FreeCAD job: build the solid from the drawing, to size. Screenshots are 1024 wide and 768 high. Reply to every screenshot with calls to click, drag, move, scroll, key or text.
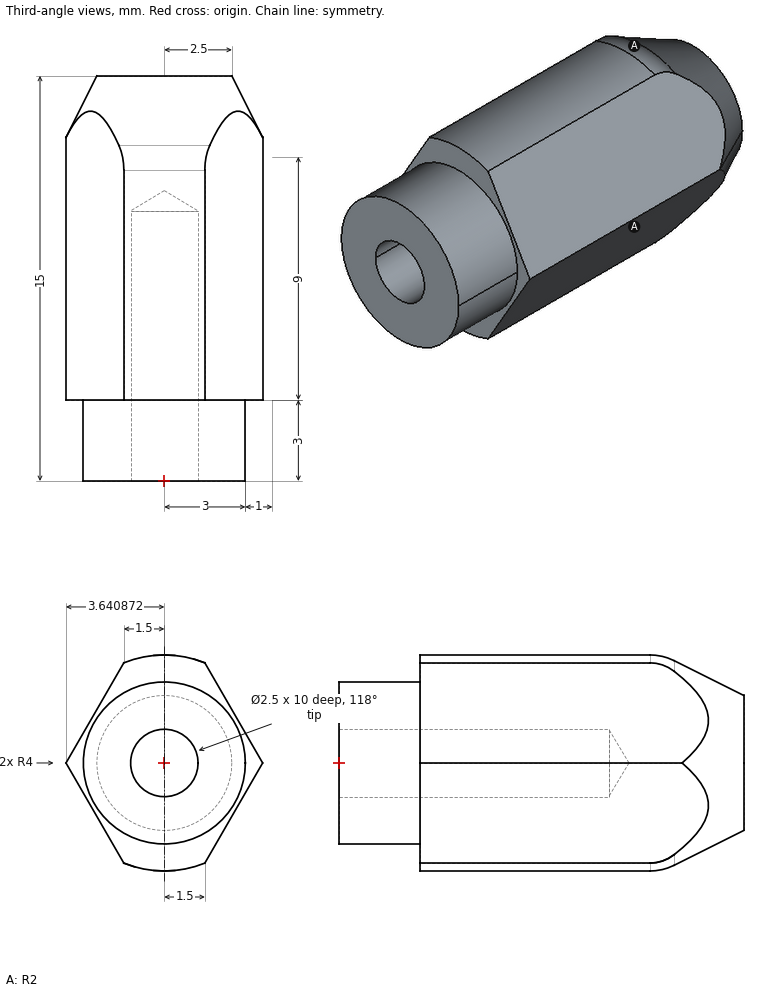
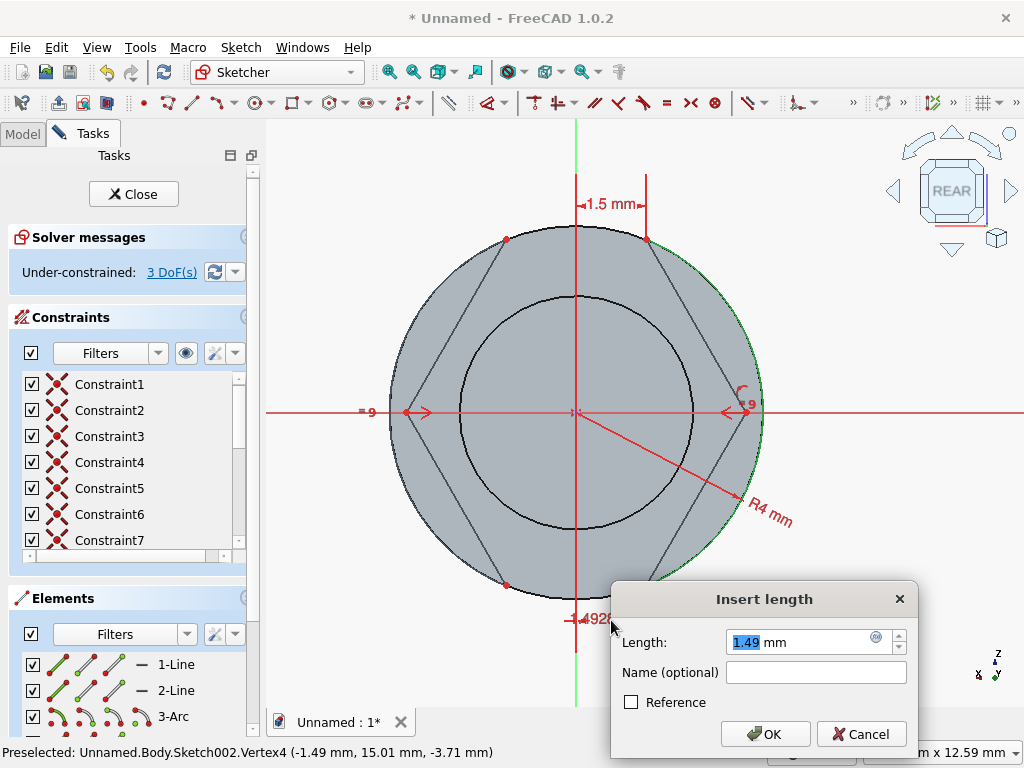
text(1.5)
key(Return)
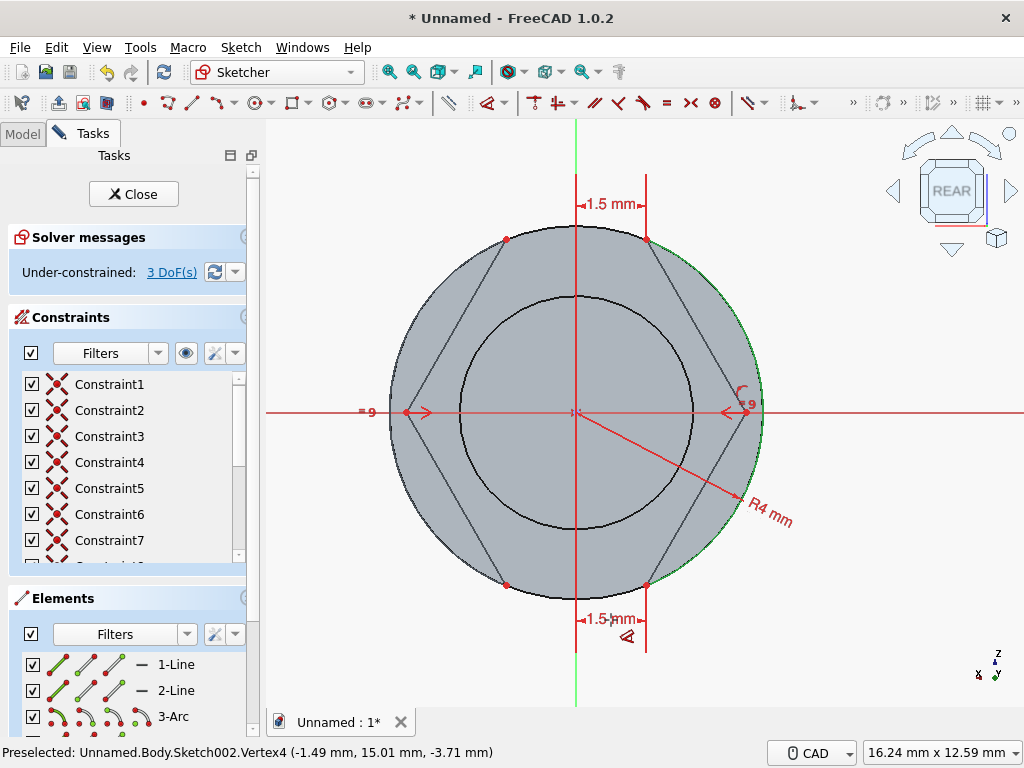
click(506, 586)
click(541, 620)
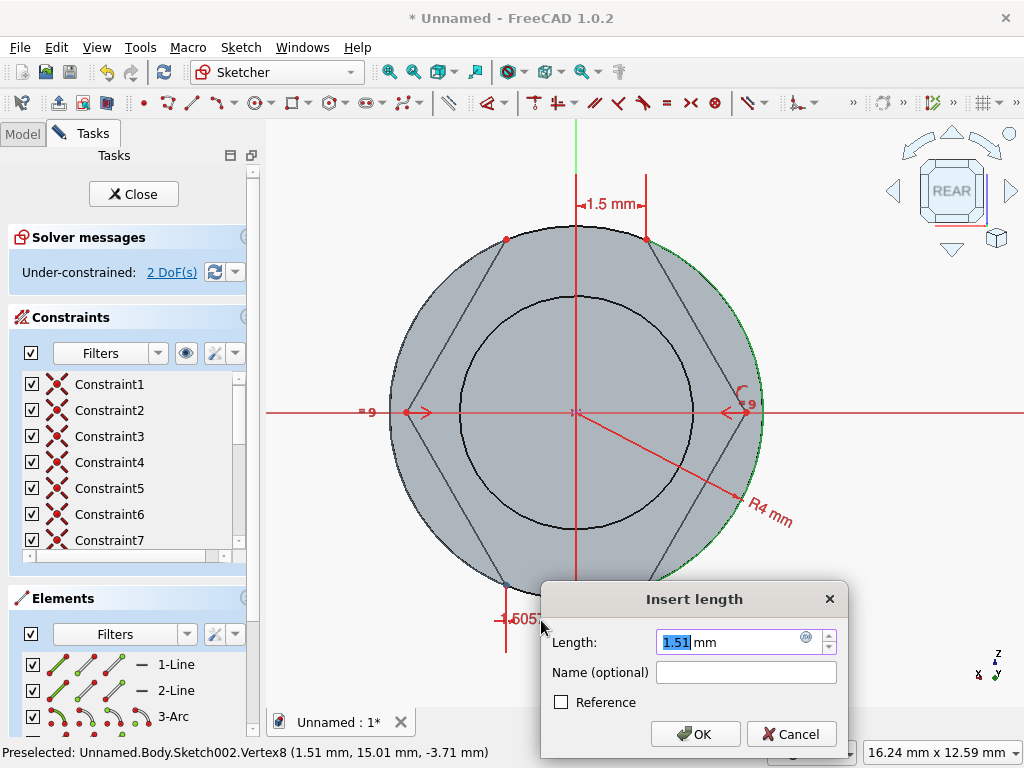
text(1.5)
key(Return)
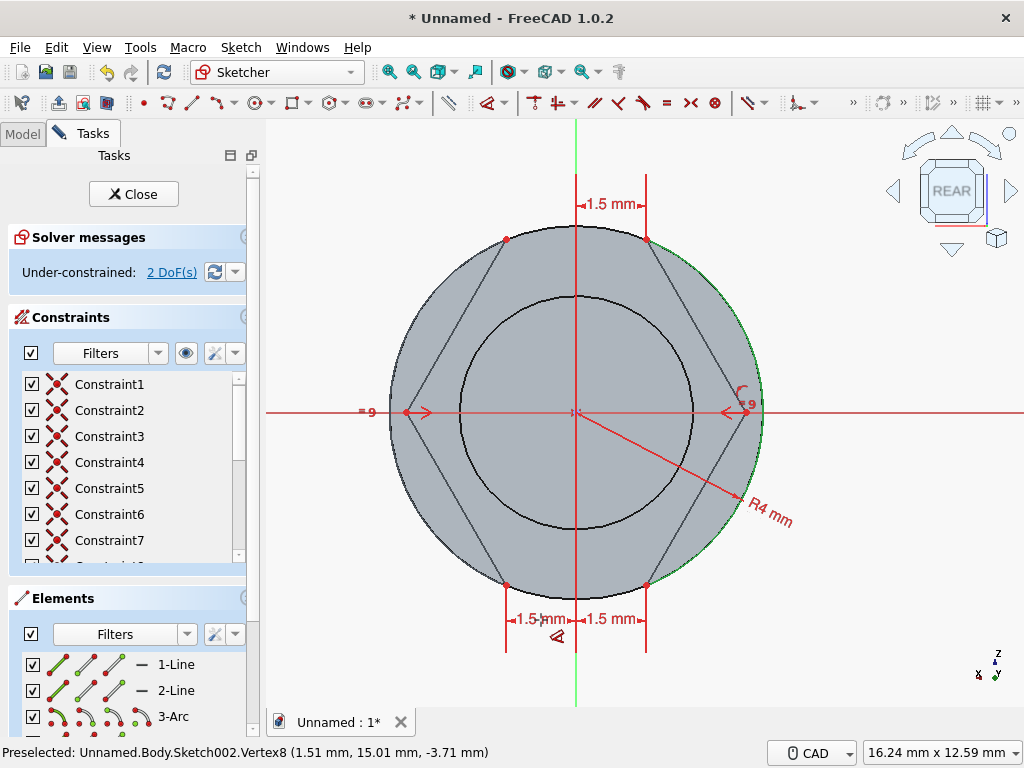
click(506, 240)
click(525, 206)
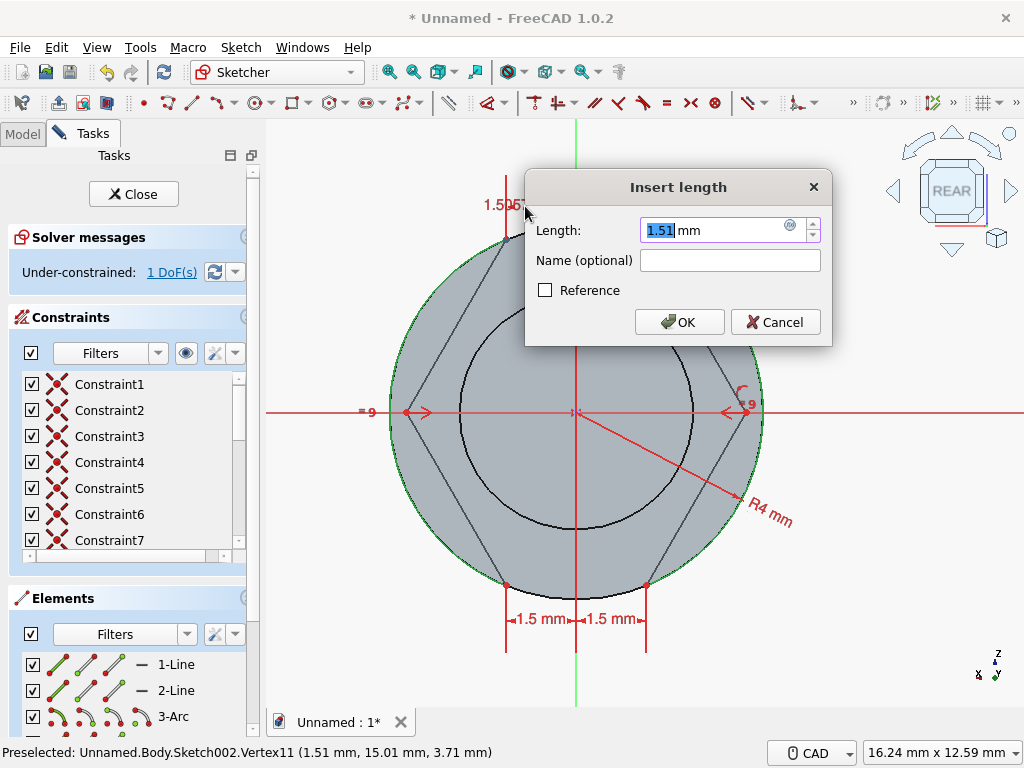
text(1.5)
key(Return)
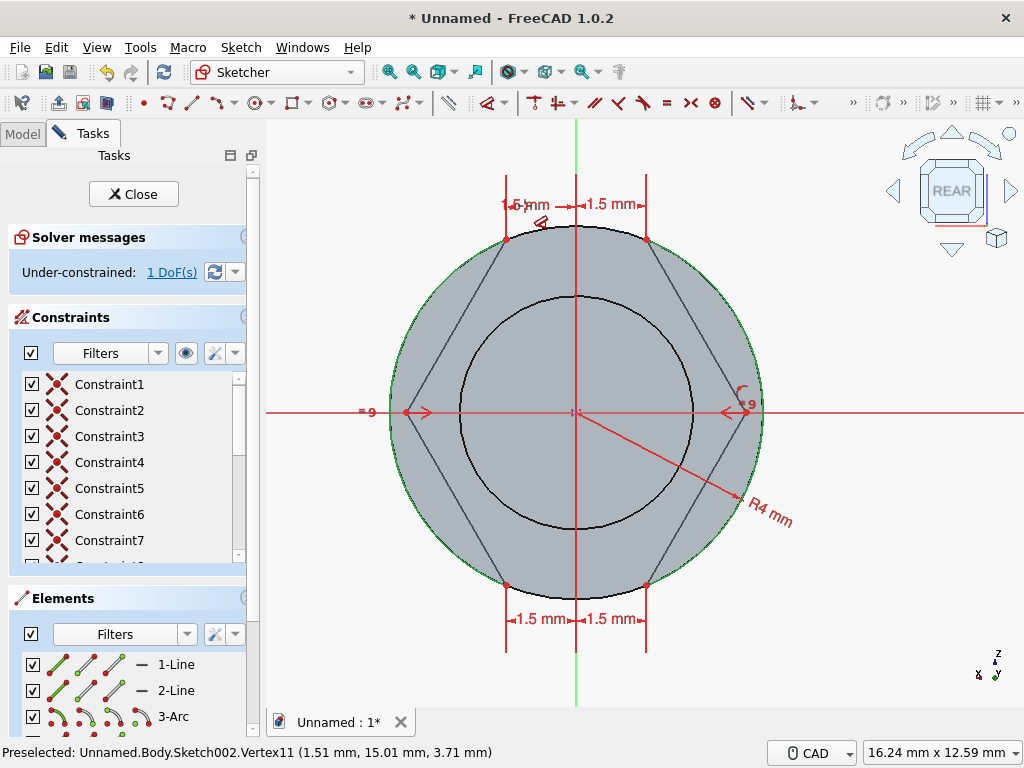
click(746, 413)
click(661, 447)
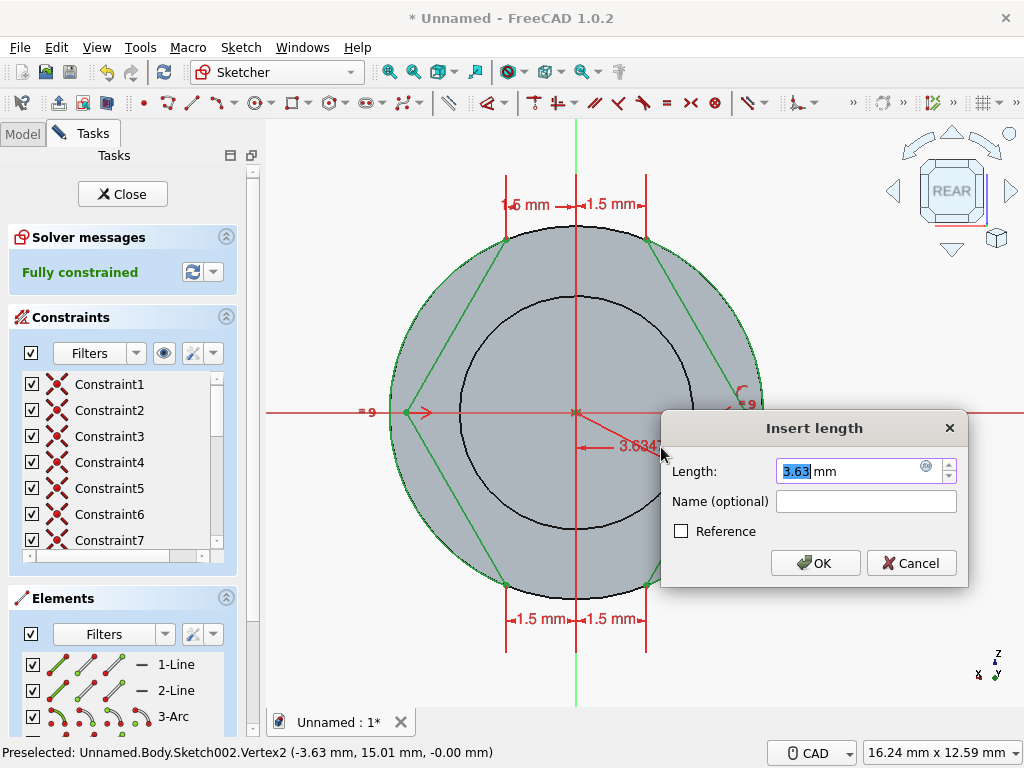
text(3.640872)
key(Return)
key(Escape)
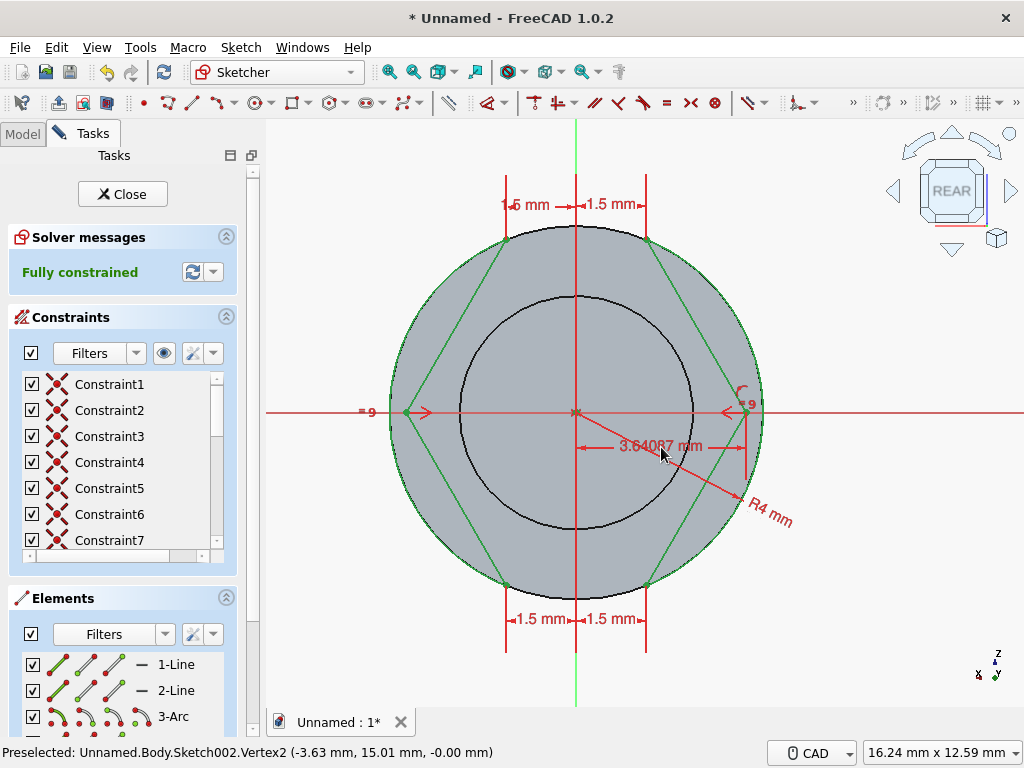
click(123, 194)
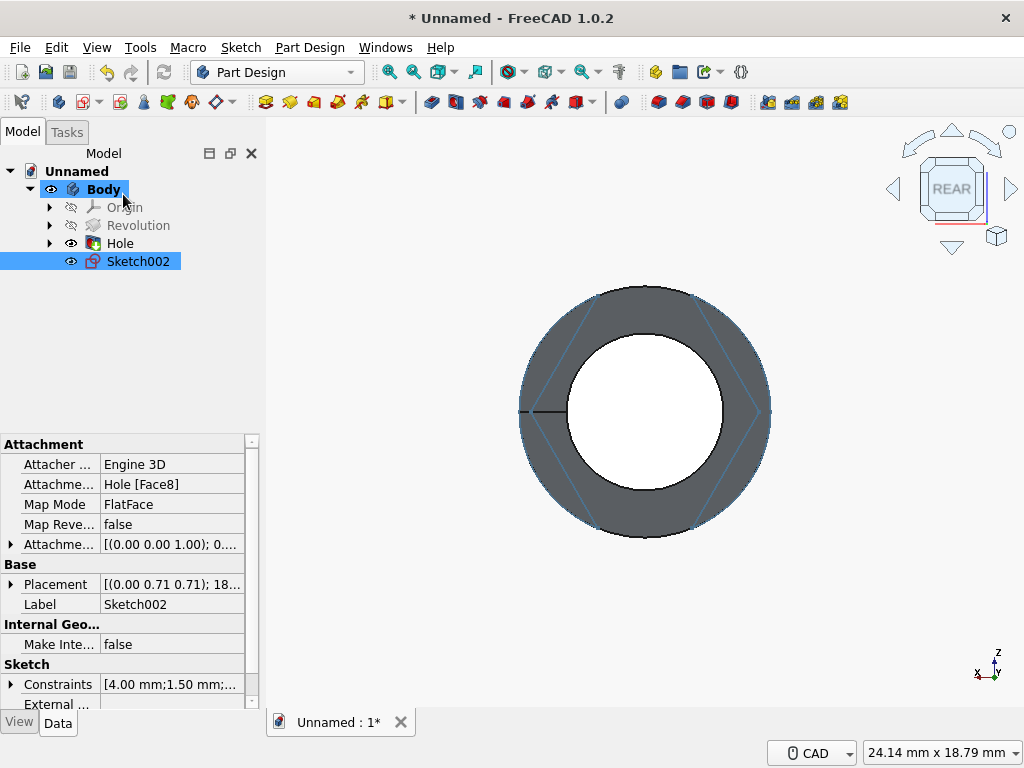
click(432, 102)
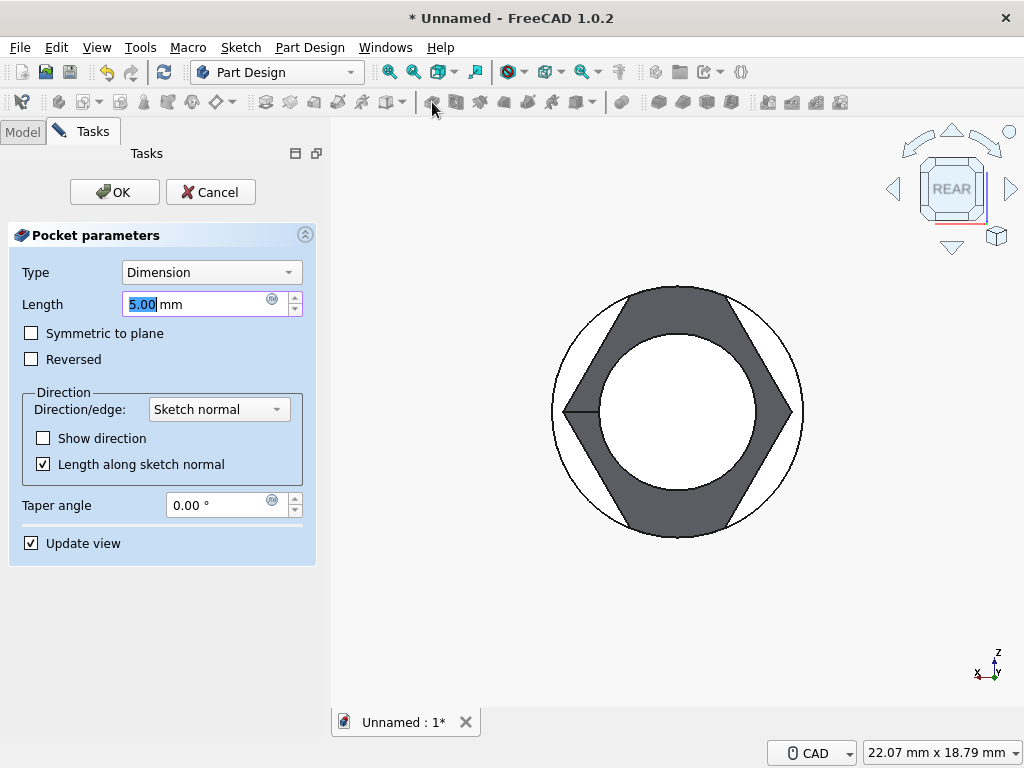
click(212, 272)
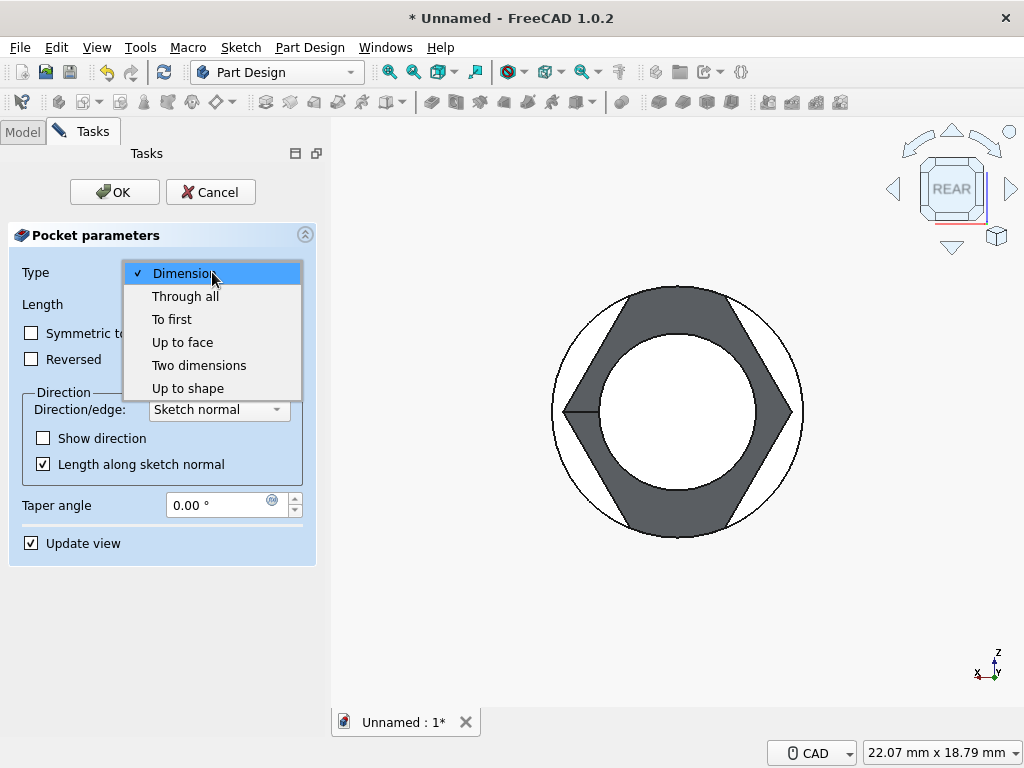
click(212, 296)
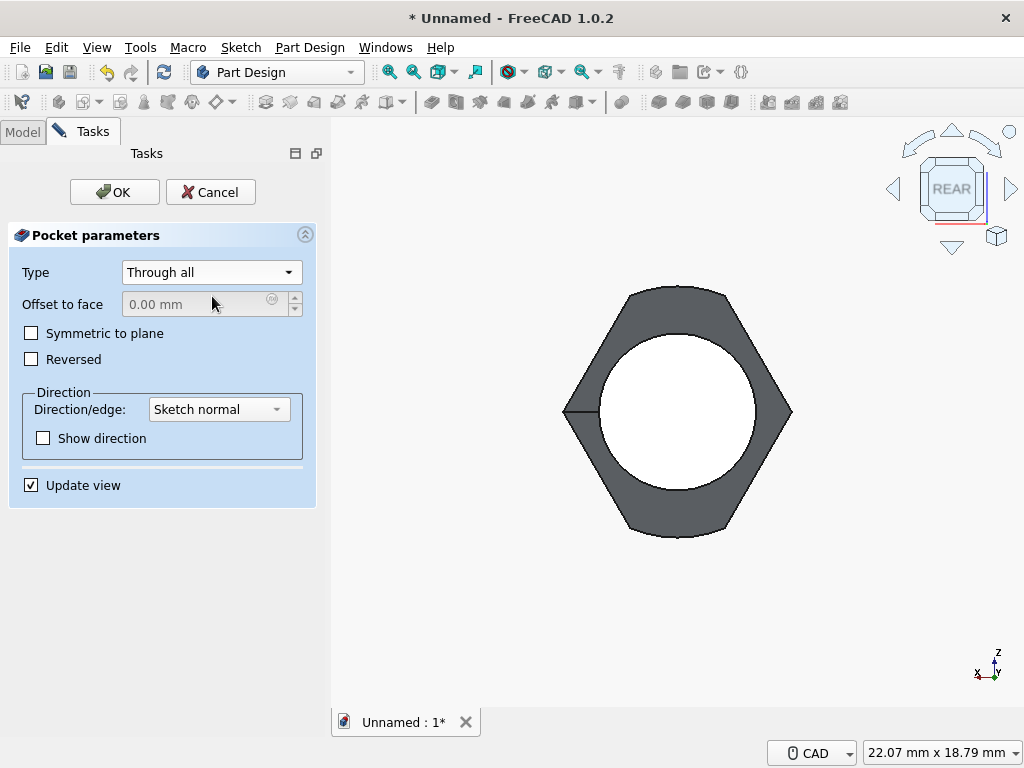
click(115, 192)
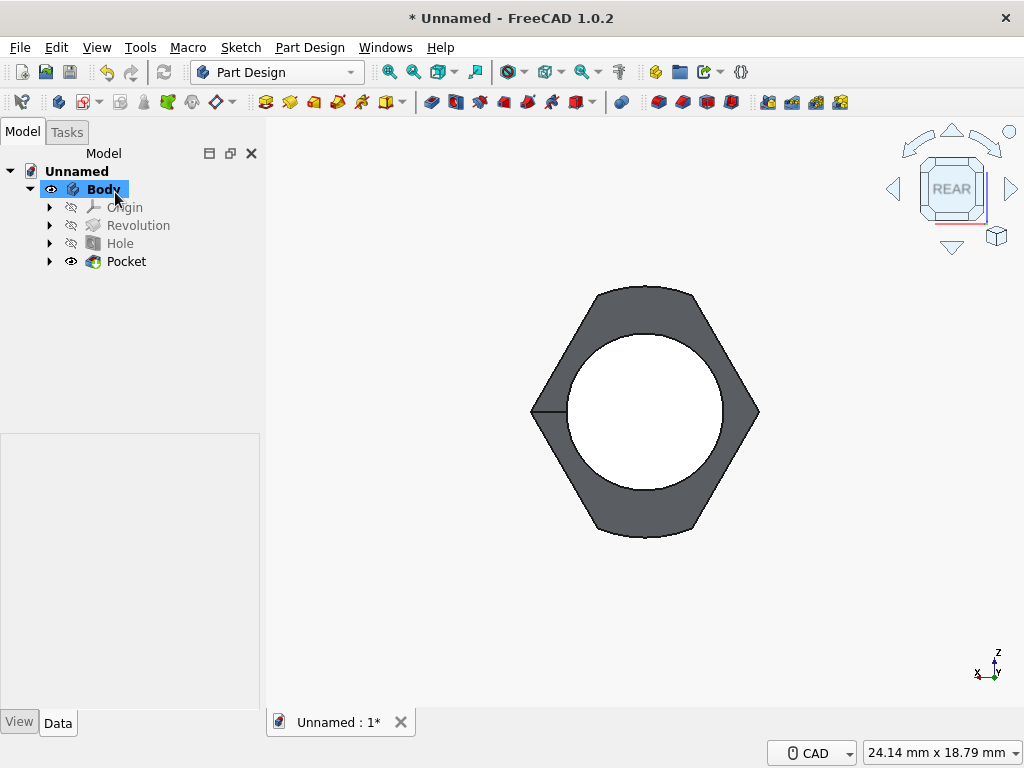
click(390, 72)